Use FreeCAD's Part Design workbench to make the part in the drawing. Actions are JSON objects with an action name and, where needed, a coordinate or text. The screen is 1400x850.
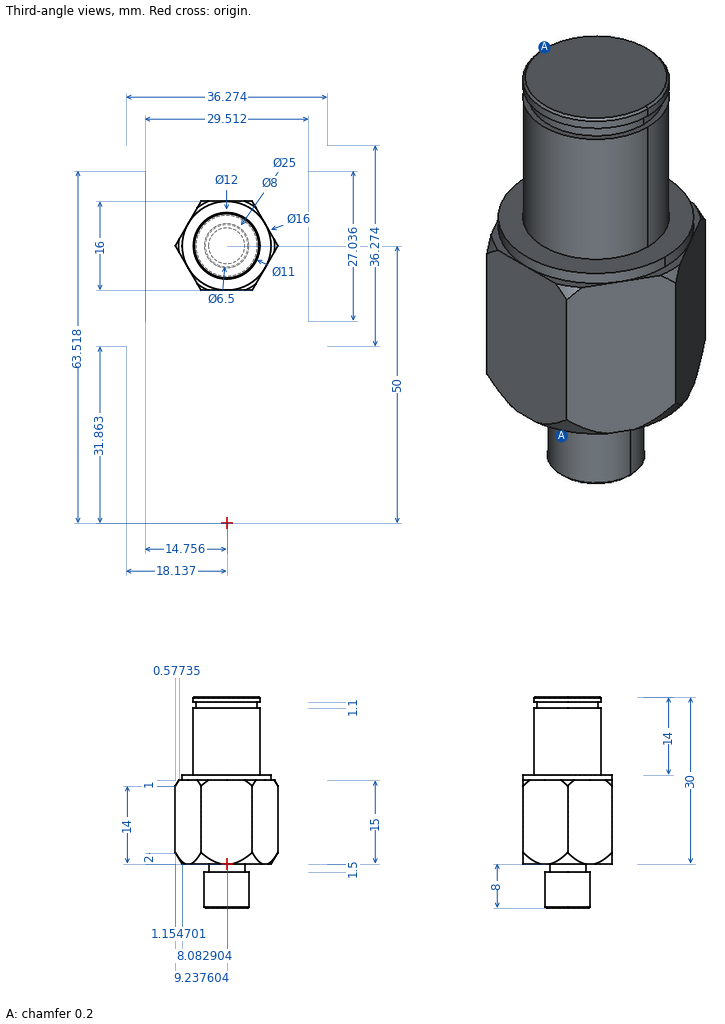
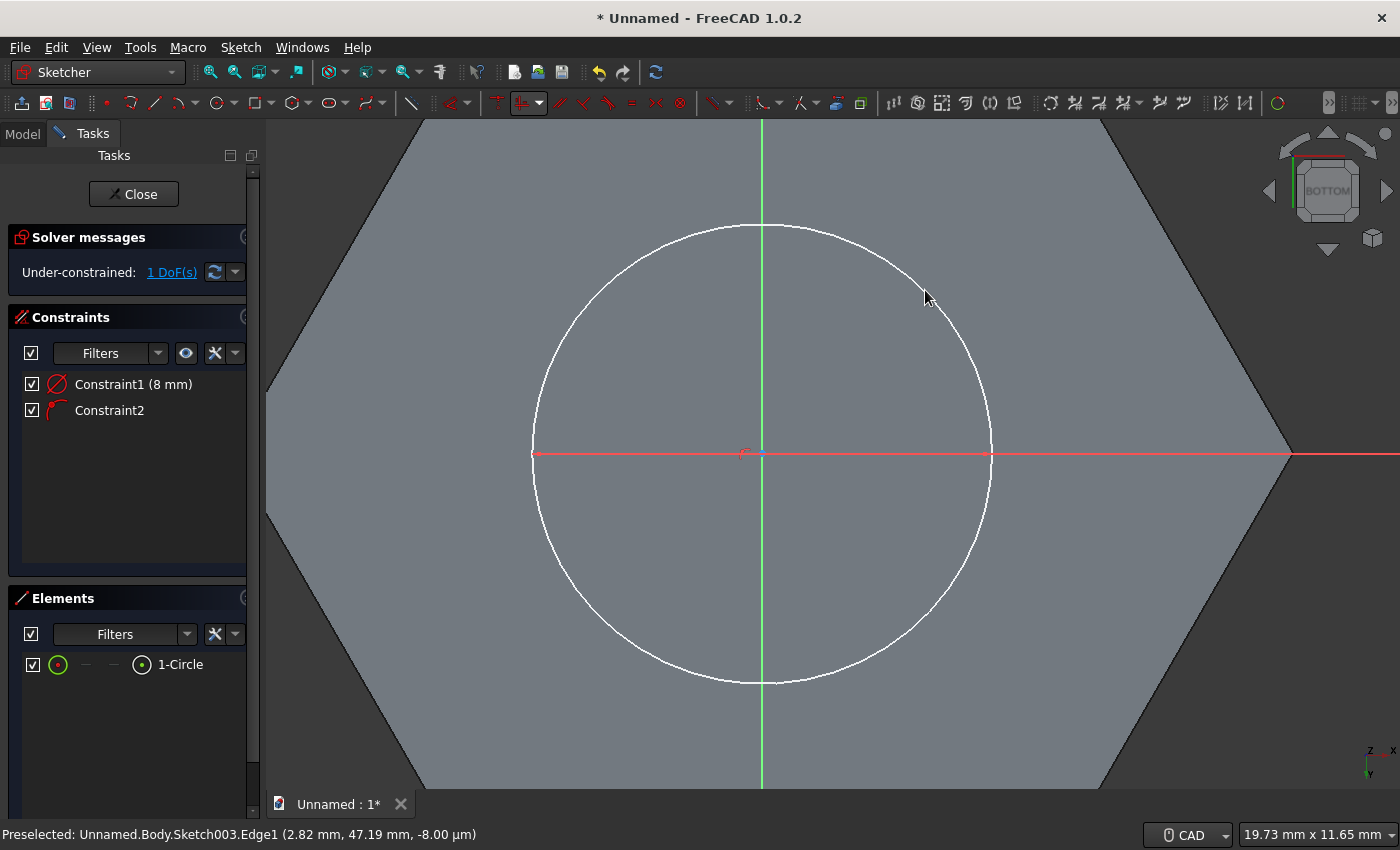
{"action": "left_click", "coordinate": [450, 104]}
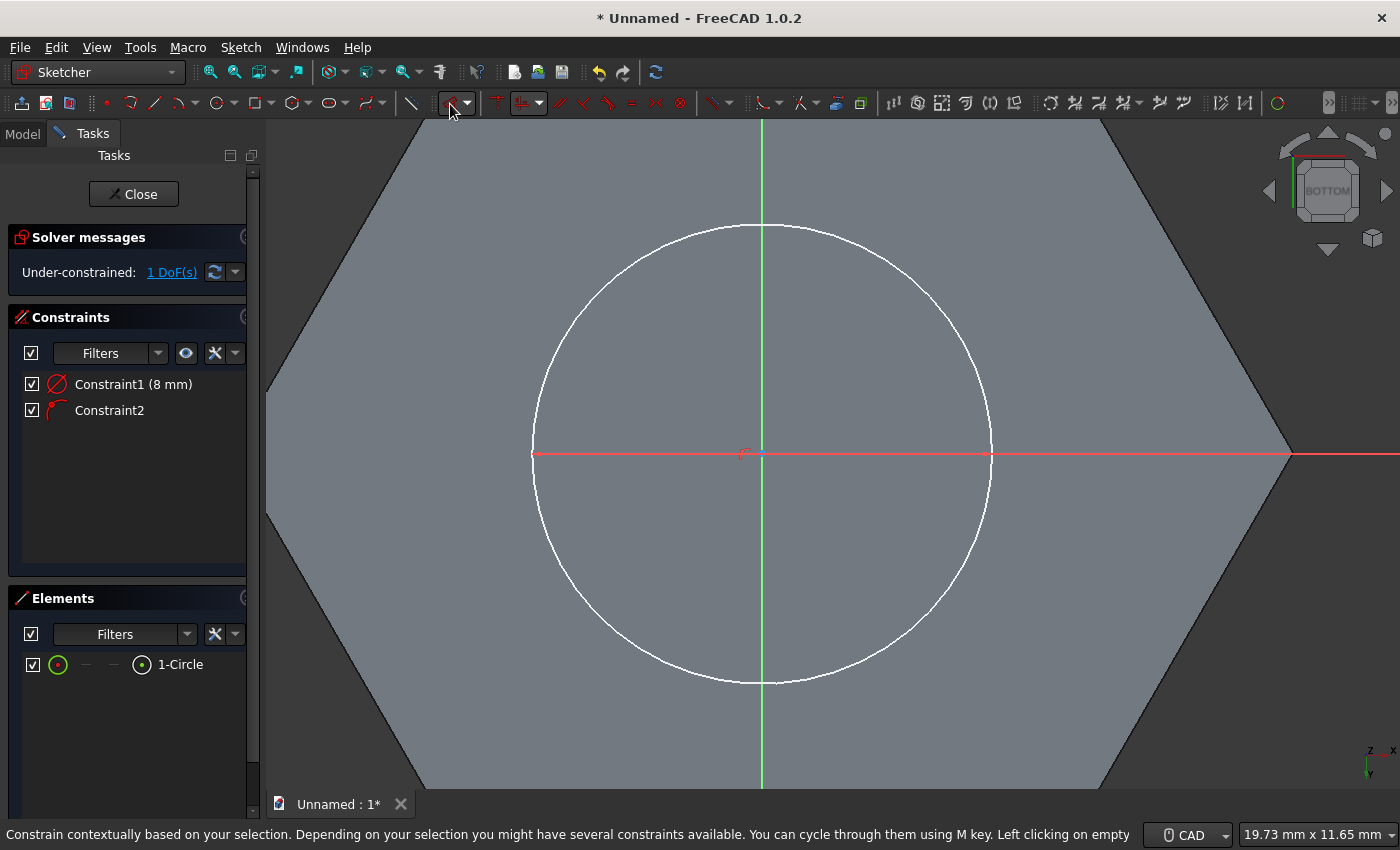
{"action": "left_click", "coordinate": [762, 454]}
{"action": "left_click", "coordinate": [796, 300]}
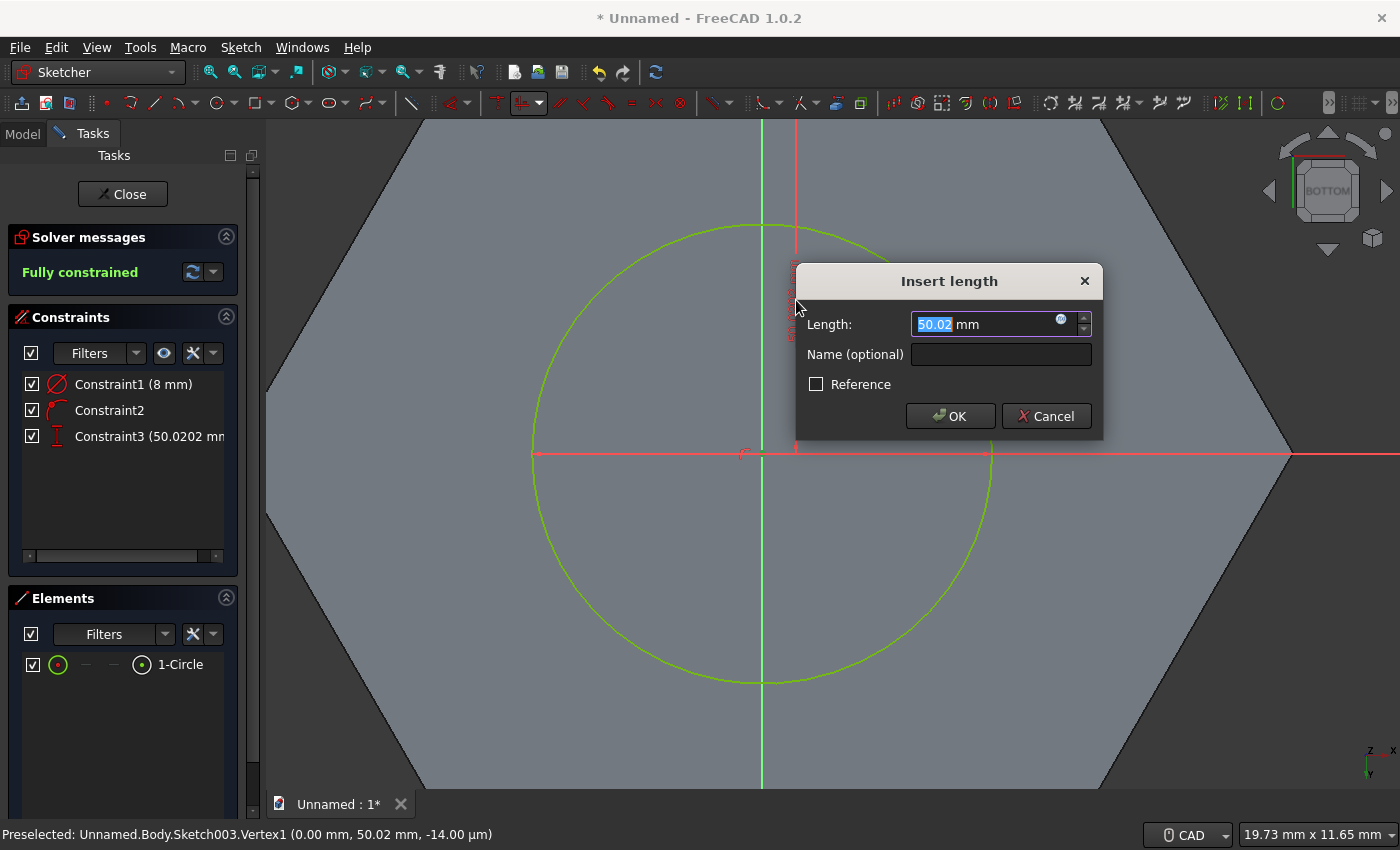
{"action": "type", "text": "50"}
{"action": "key", "text": "Return"}
{"action": "key", "text": "Escape"}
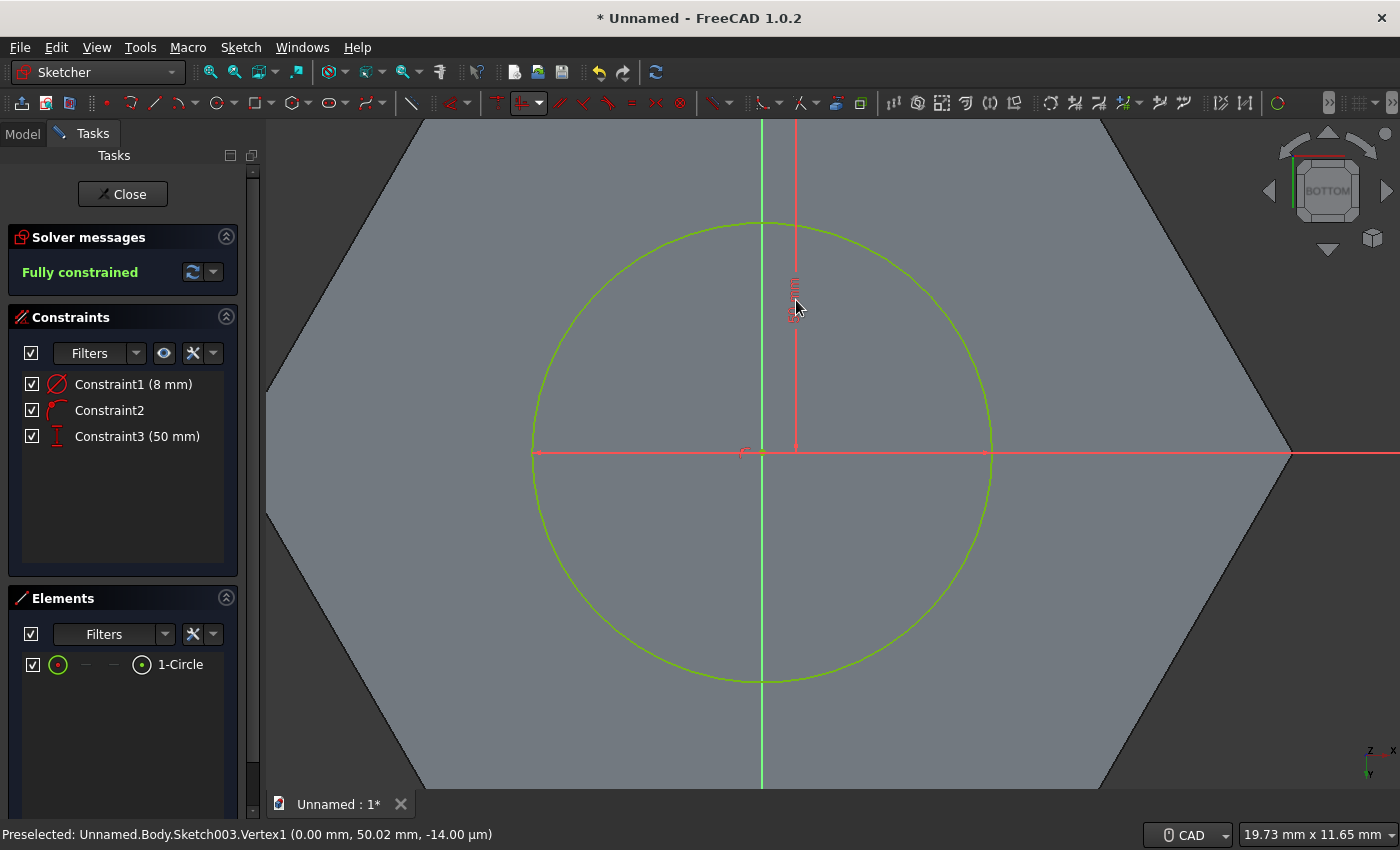
{"action": "left_click", "coordinate": [123, 194]}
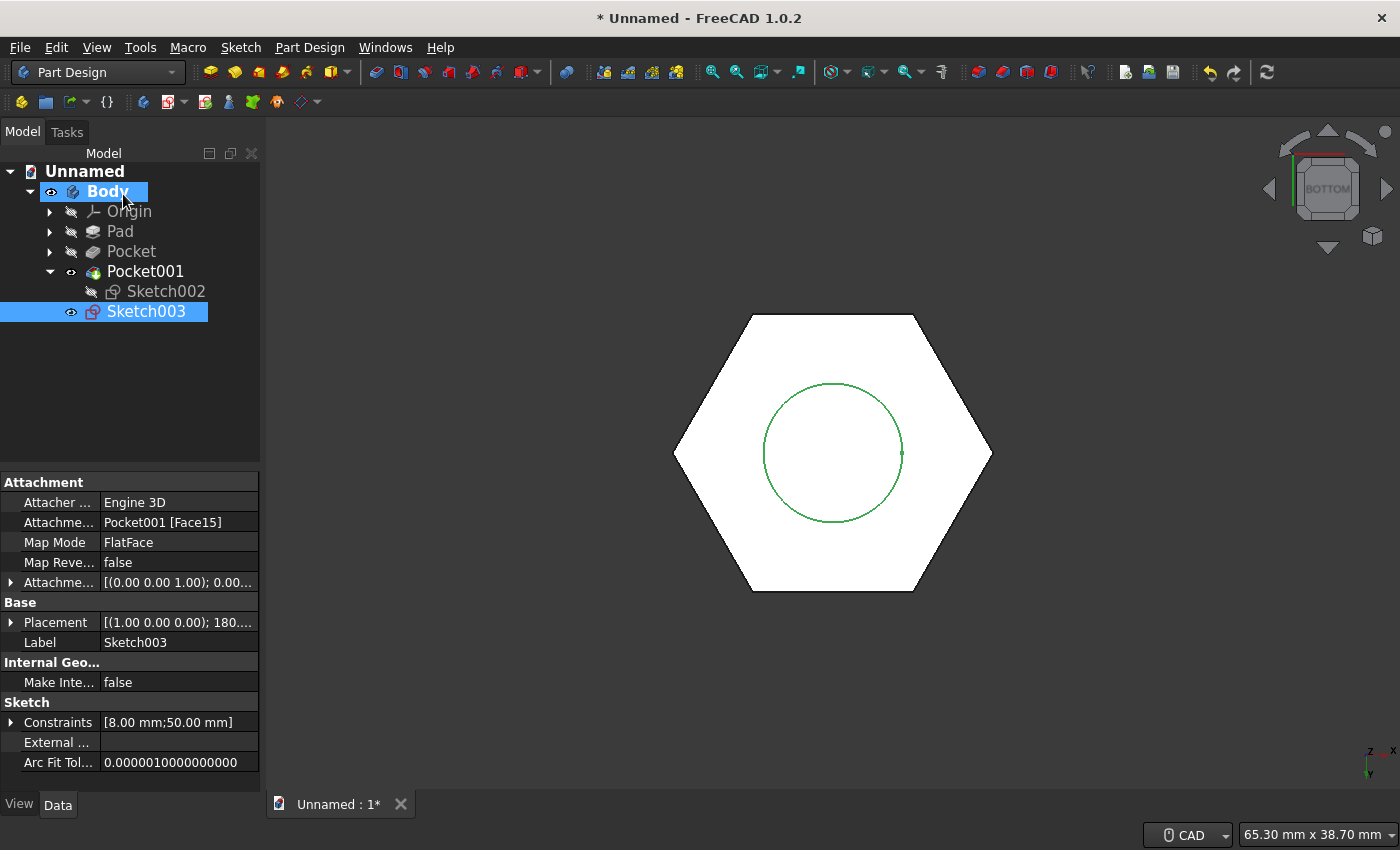
{"action": "left_click", "coordinate": [212, 72]}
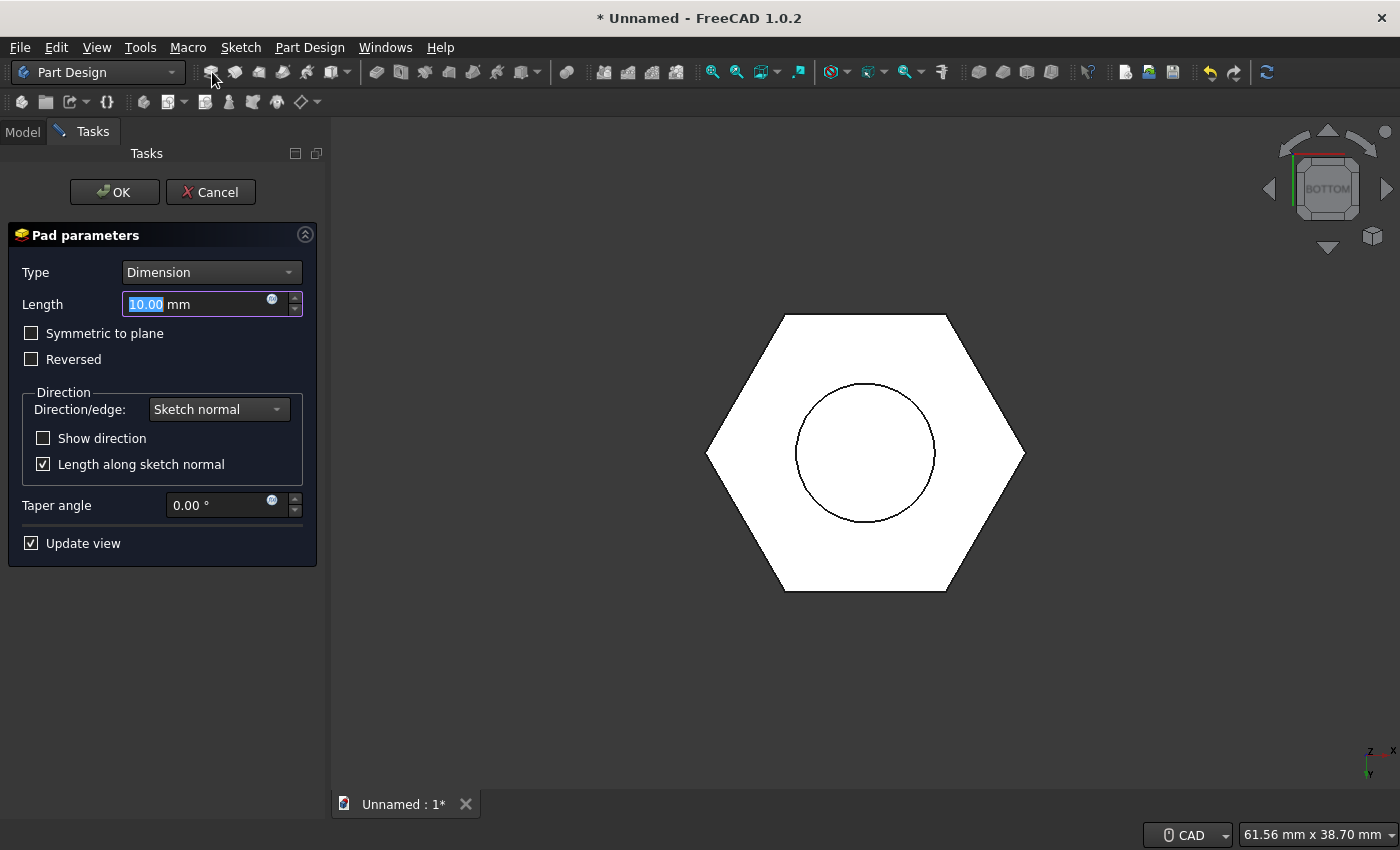
{"action": "type", "text": "8"}
{"action": "key", "text": "Tab"}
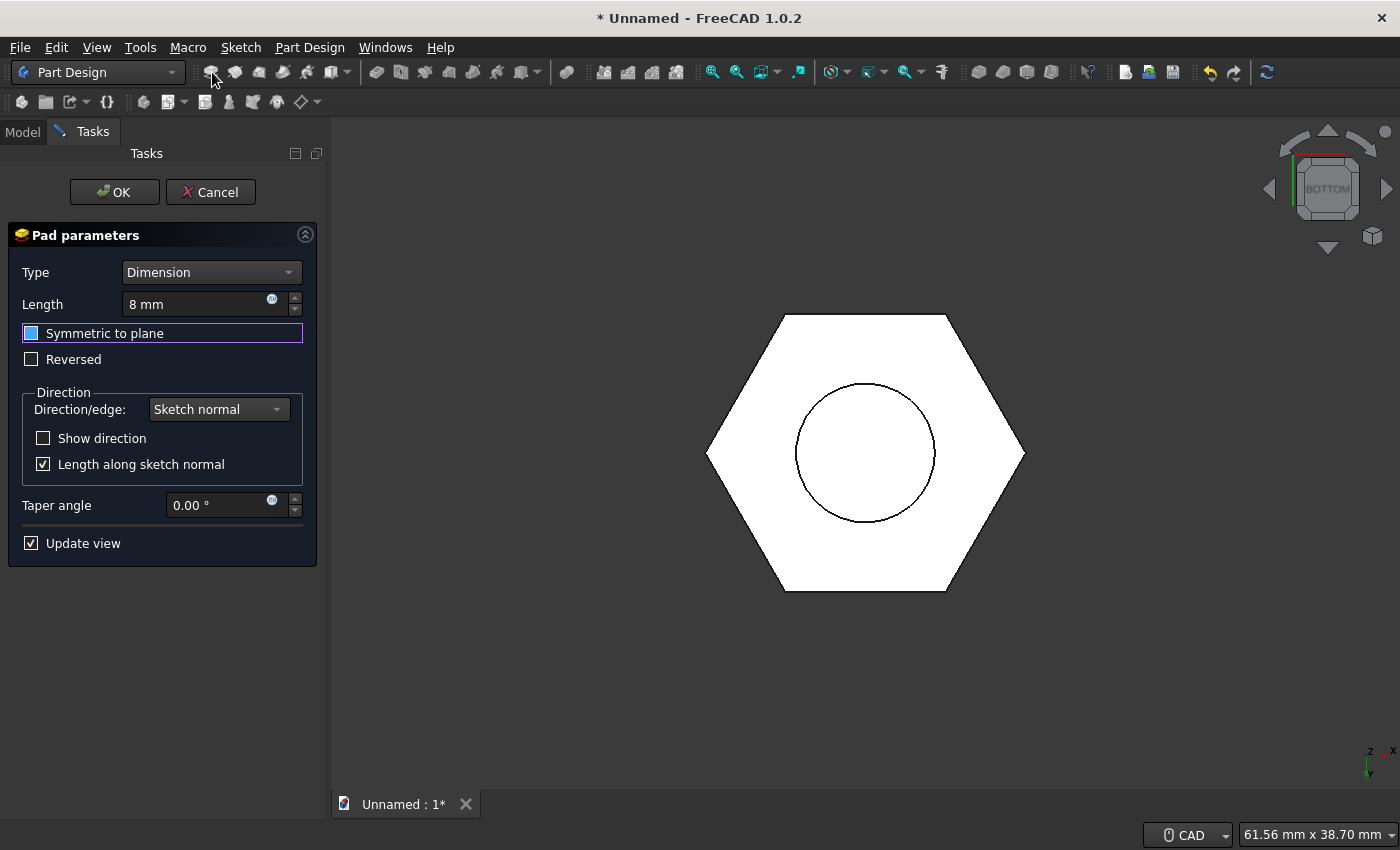
{"action": "left_click", "coordinate": [115, 192]}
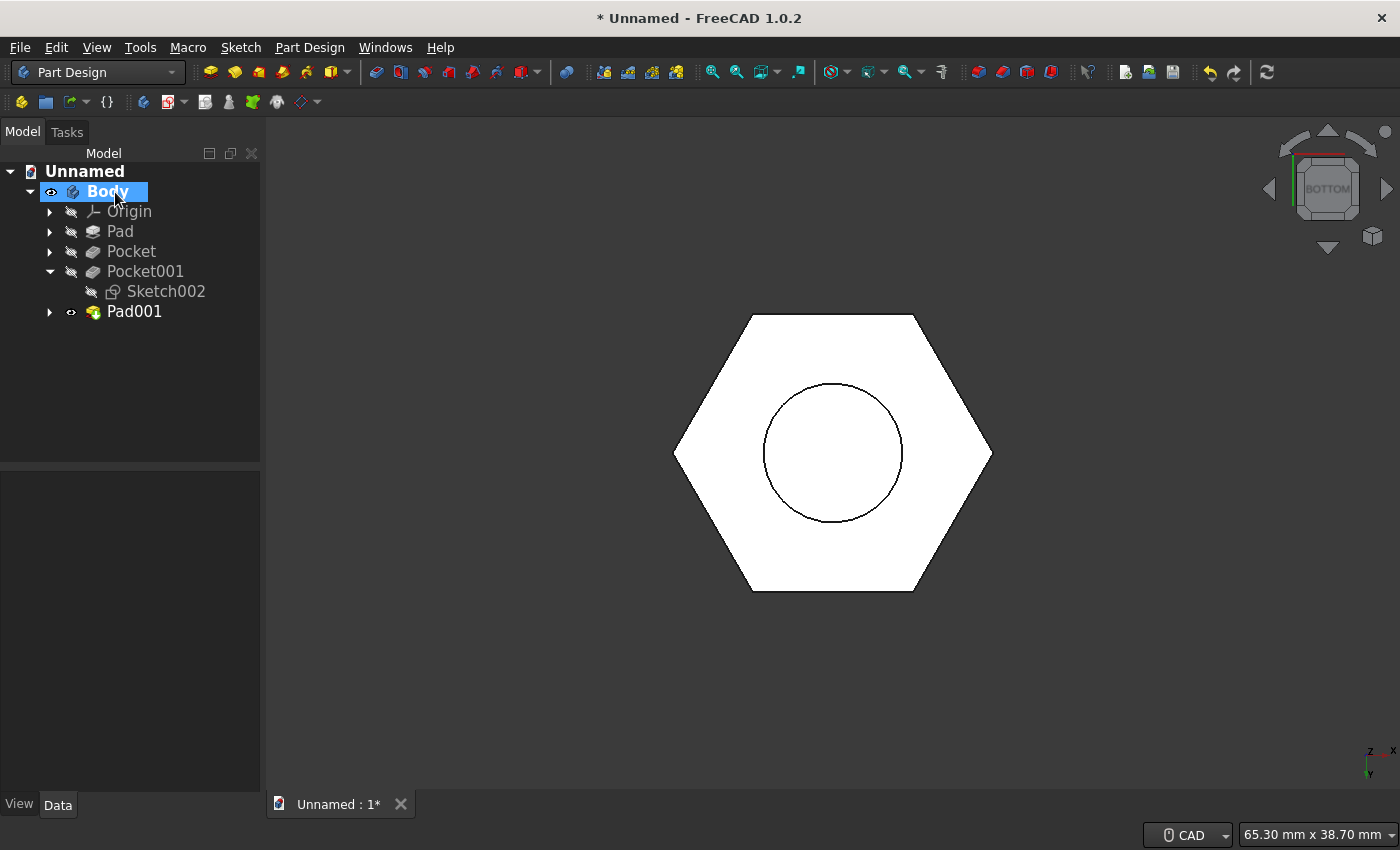
{"action": "left_click", "coordinate": [714, 72]}